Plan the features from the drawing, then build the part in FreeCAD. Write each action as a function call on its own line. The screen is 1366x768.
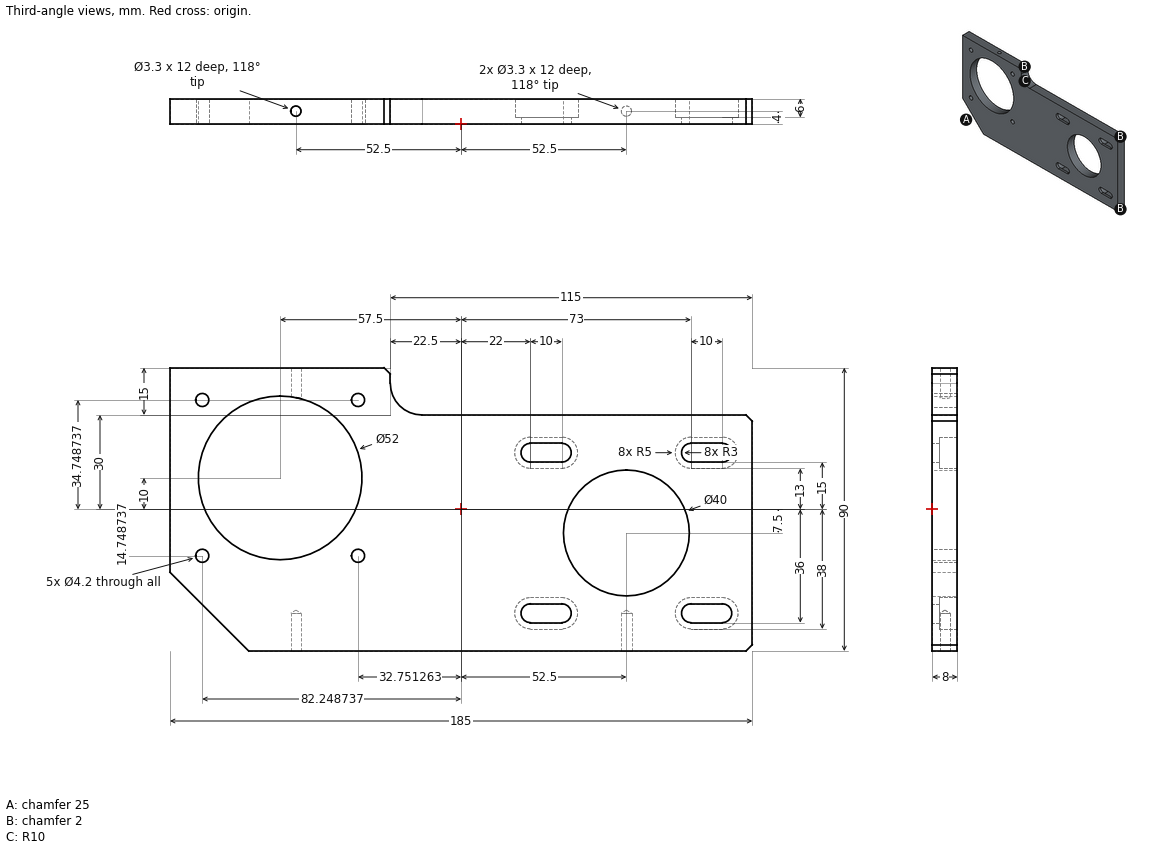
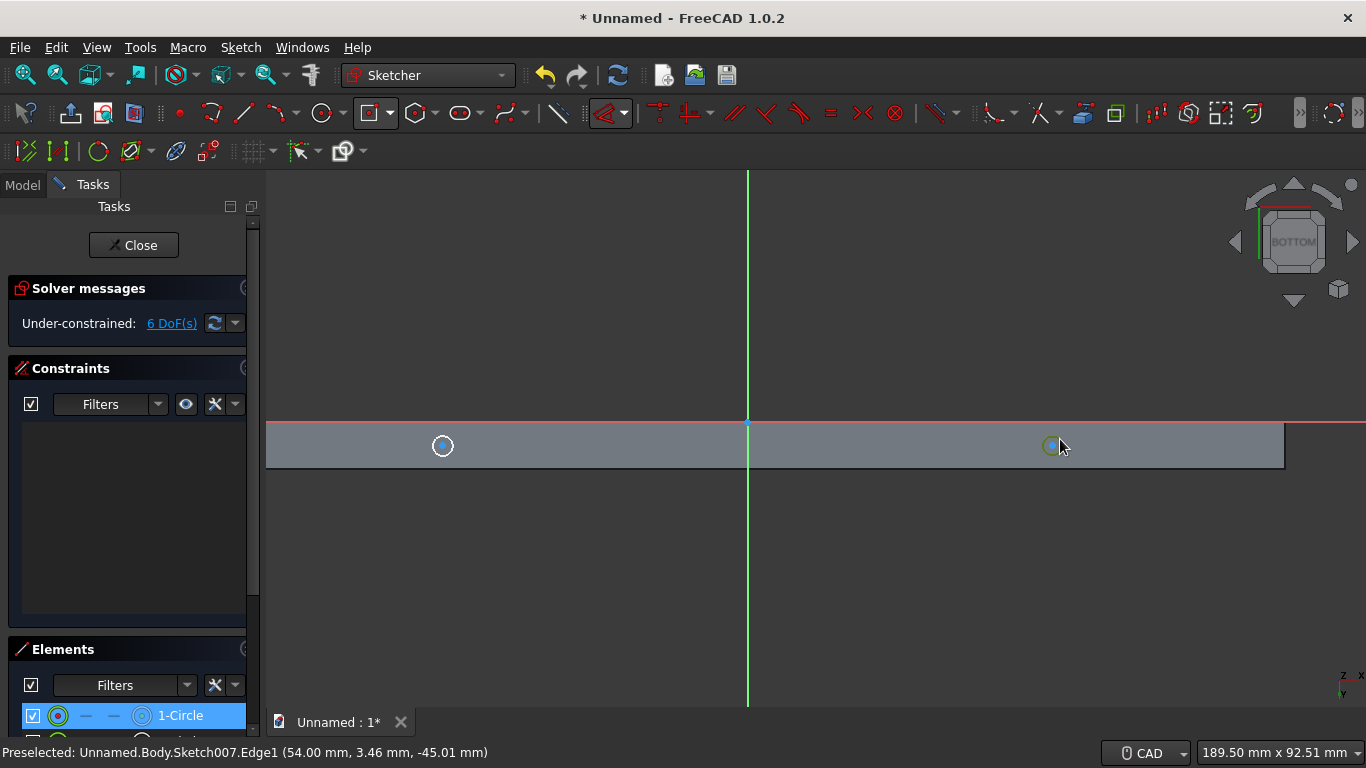
scroll(450, 439, up, 2)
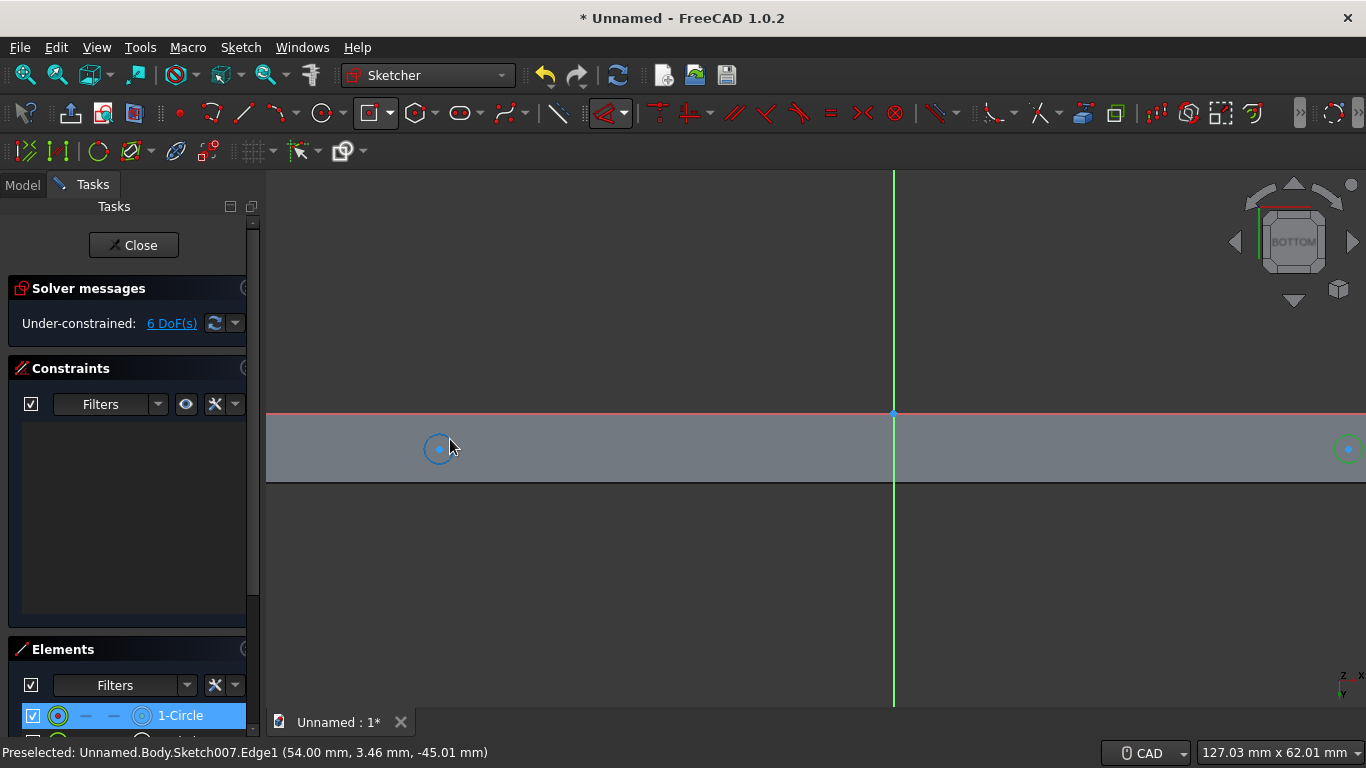
click(450, 439)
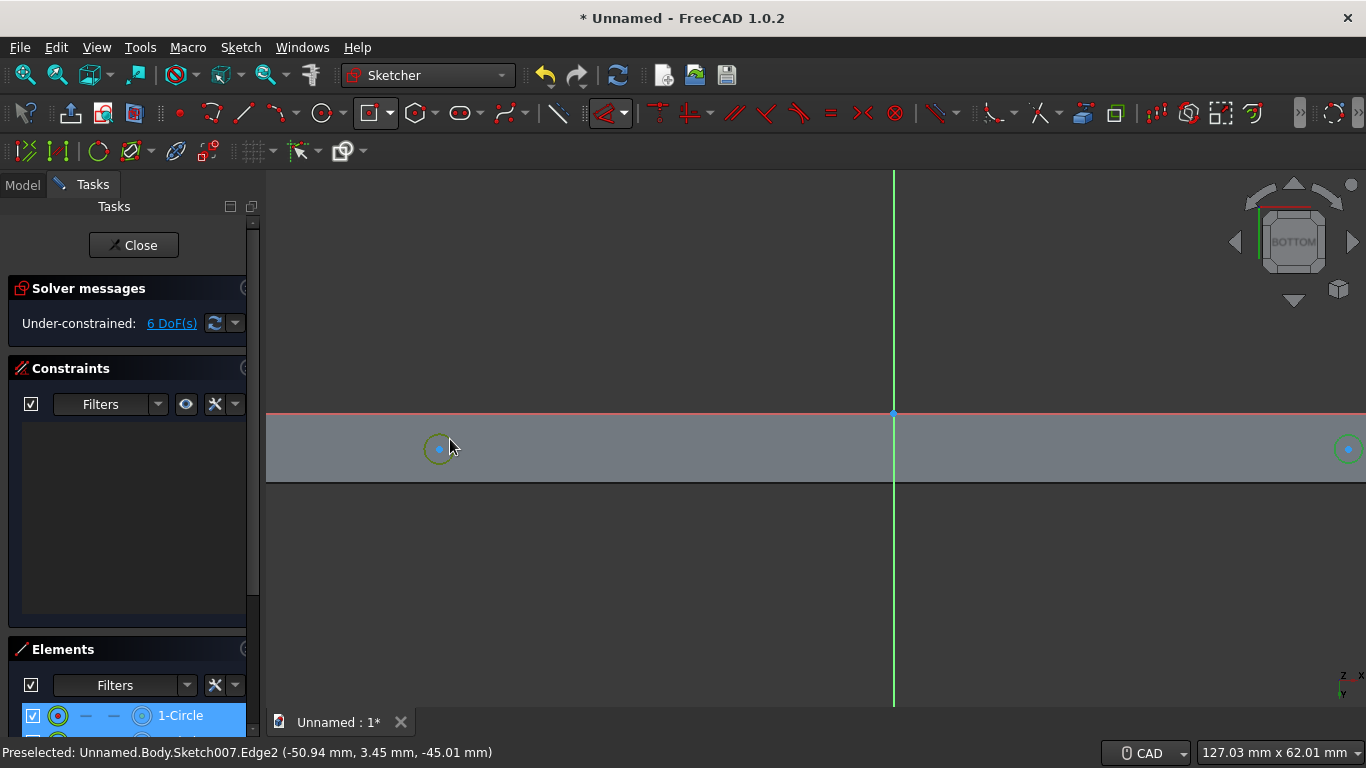
click(832, 114)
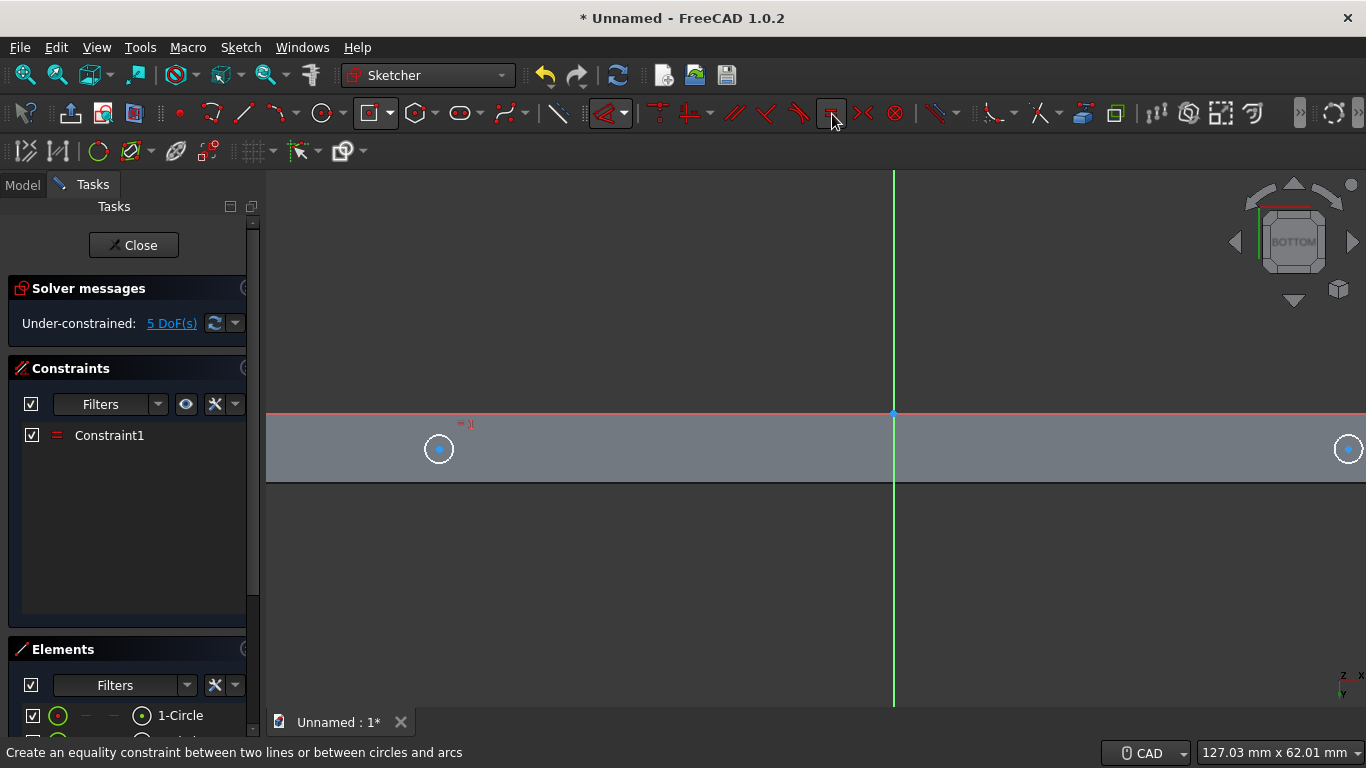
scroll(450, 439, down, 2)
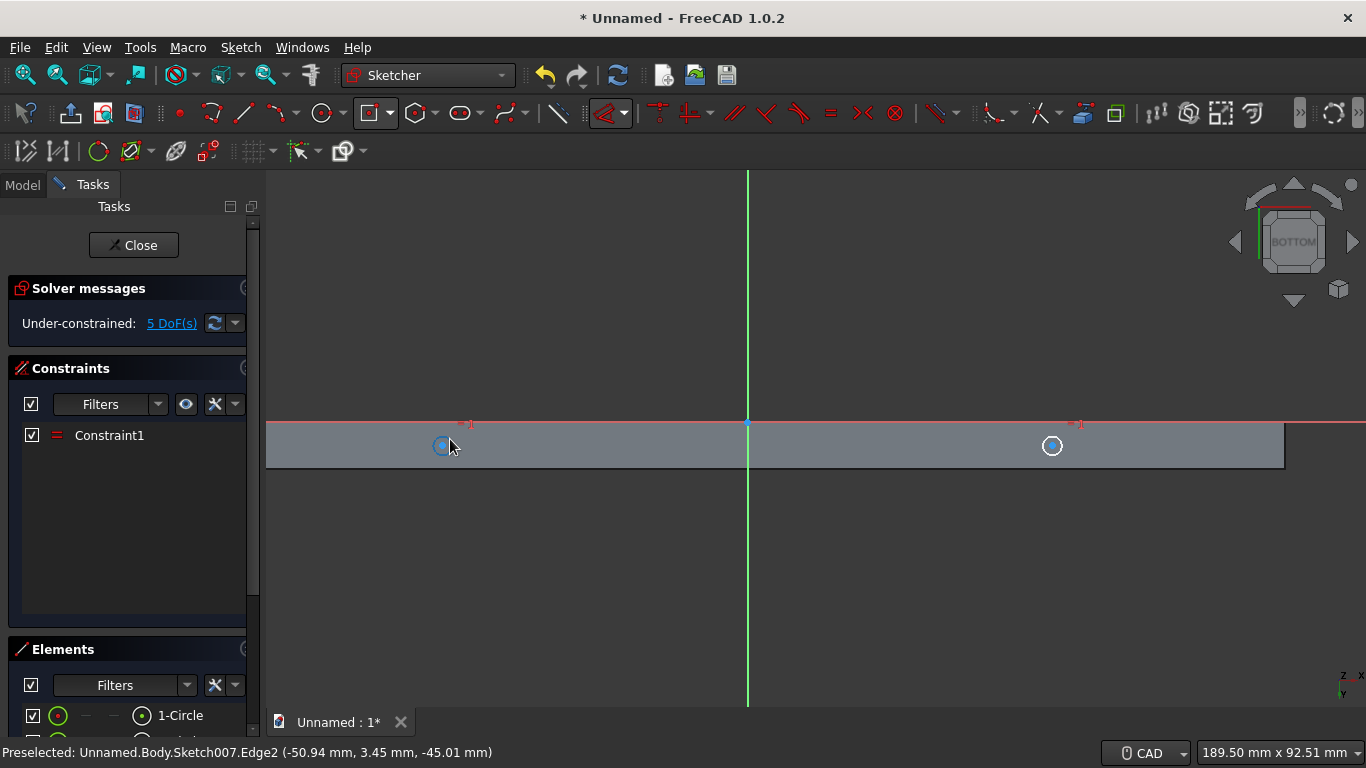
click(1052, 446)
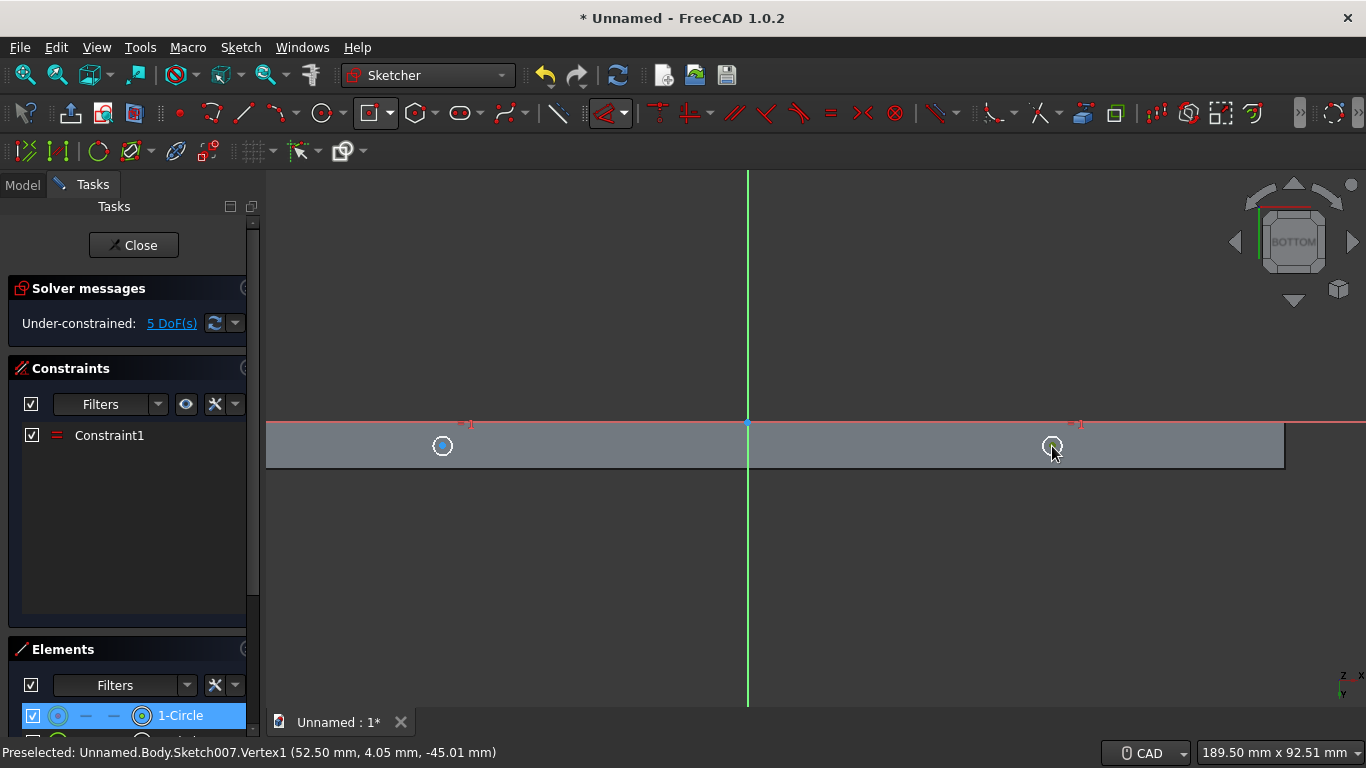
click(443, 446)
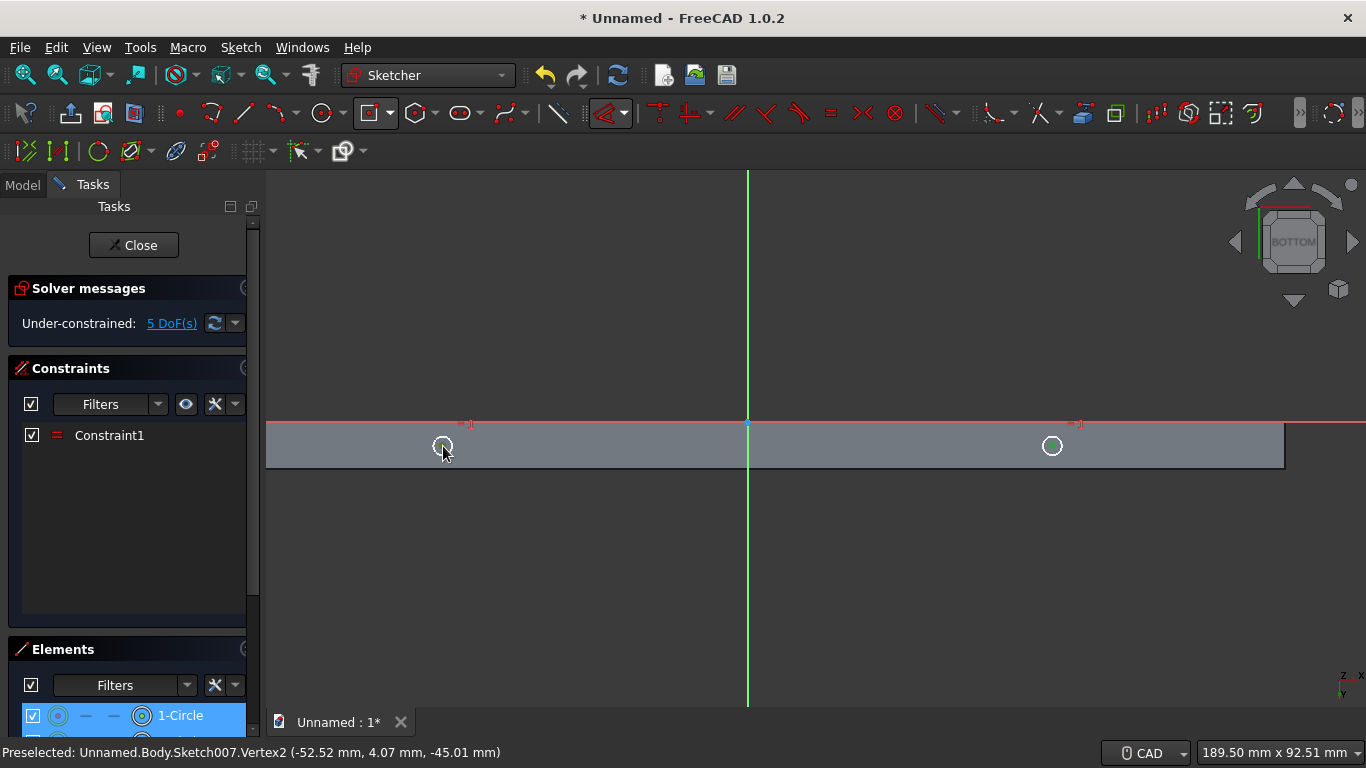
key(h)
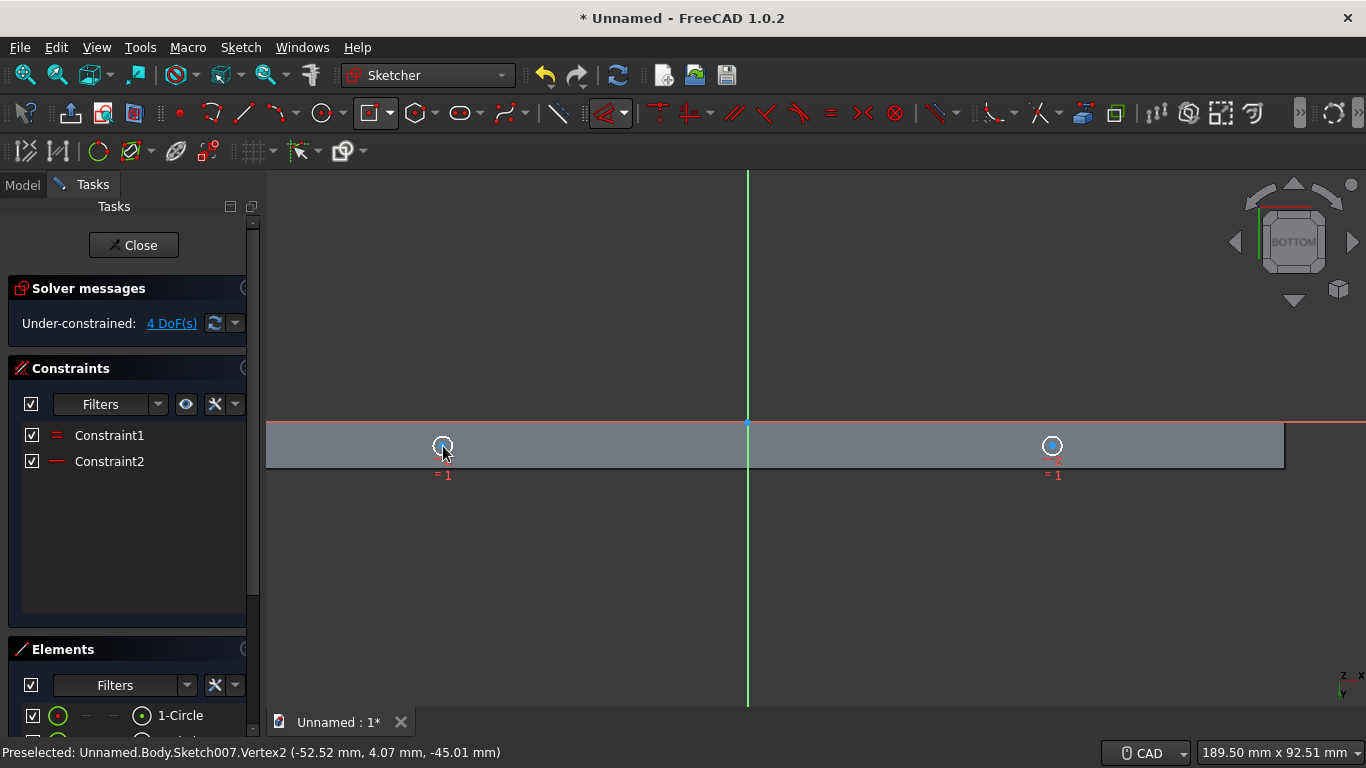
scroll(1059, 439, up, 4)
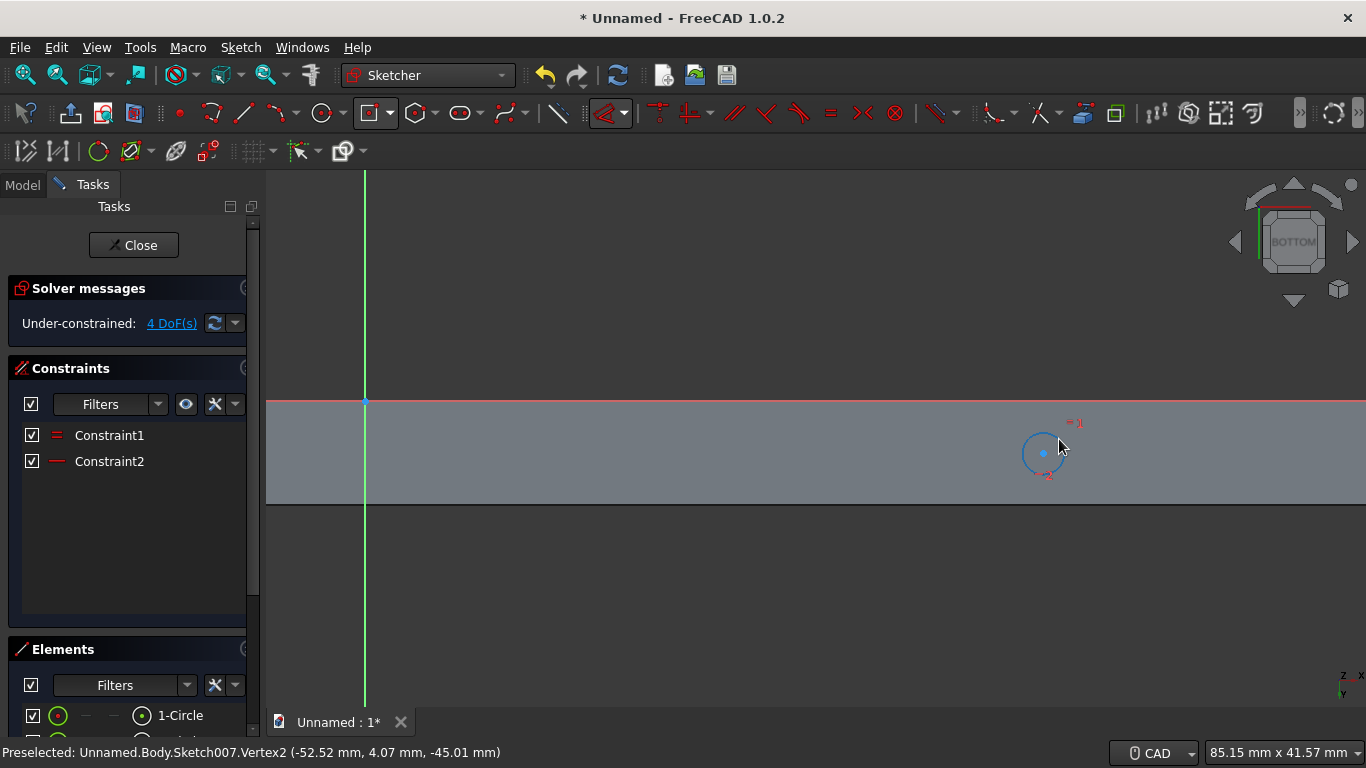
click(1058, 439)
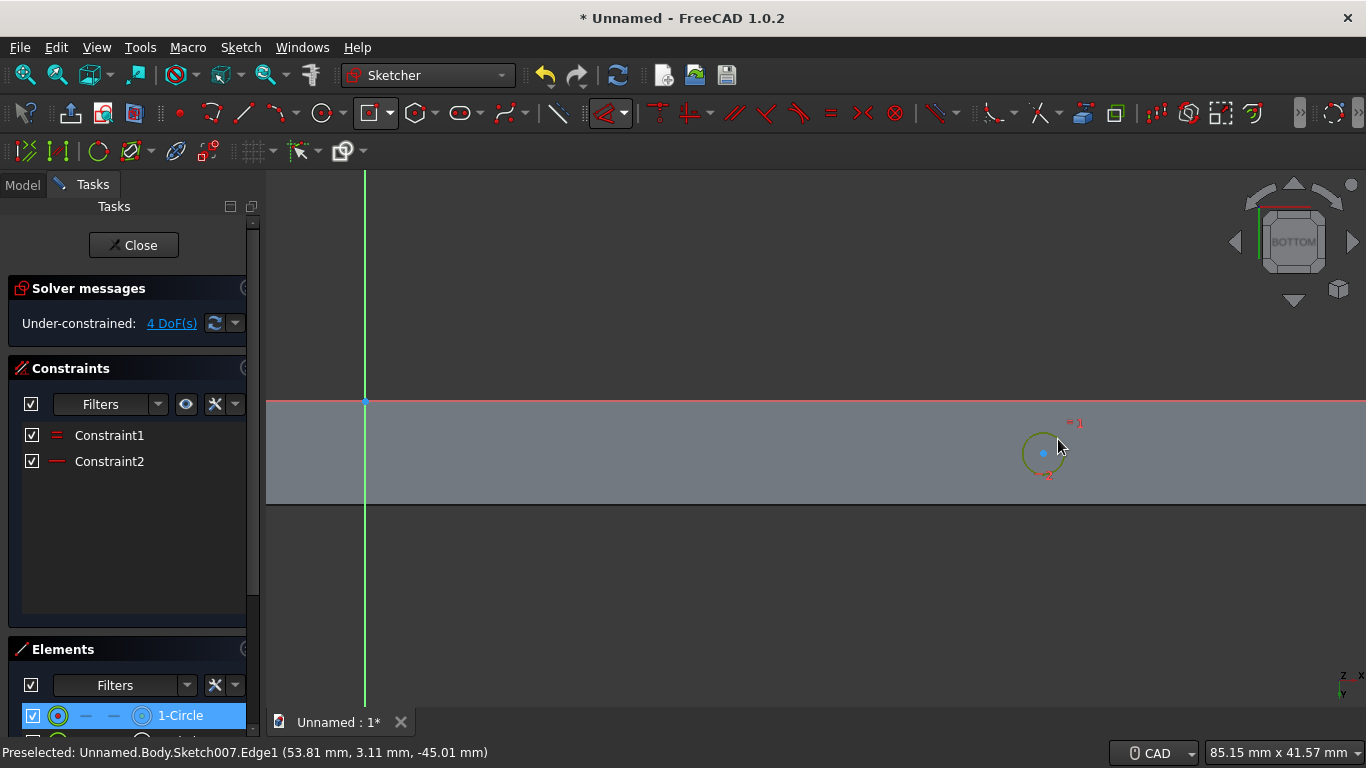
key(k)
key(o)